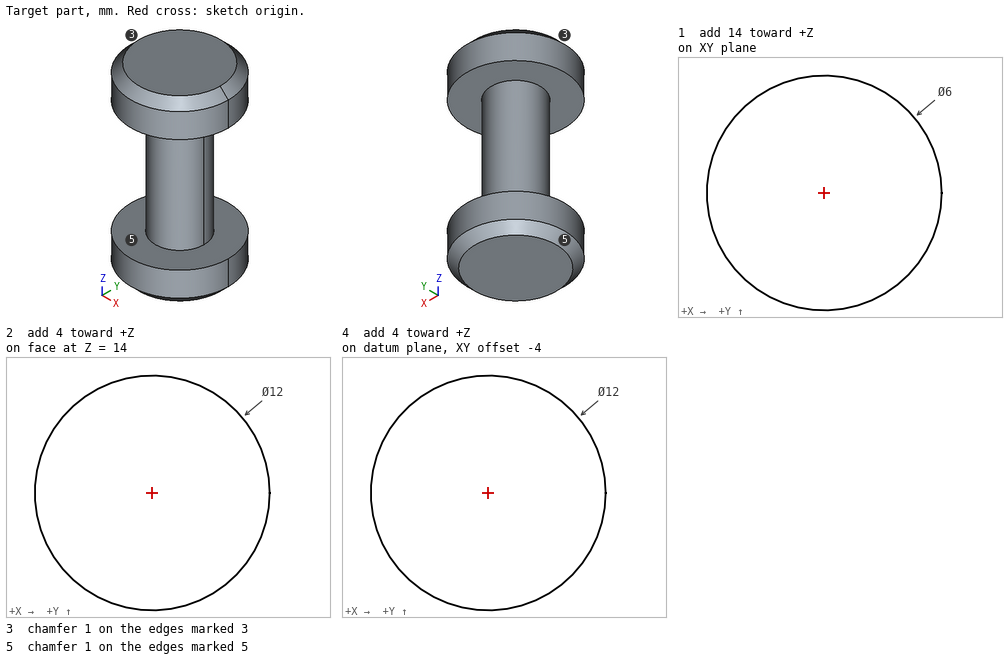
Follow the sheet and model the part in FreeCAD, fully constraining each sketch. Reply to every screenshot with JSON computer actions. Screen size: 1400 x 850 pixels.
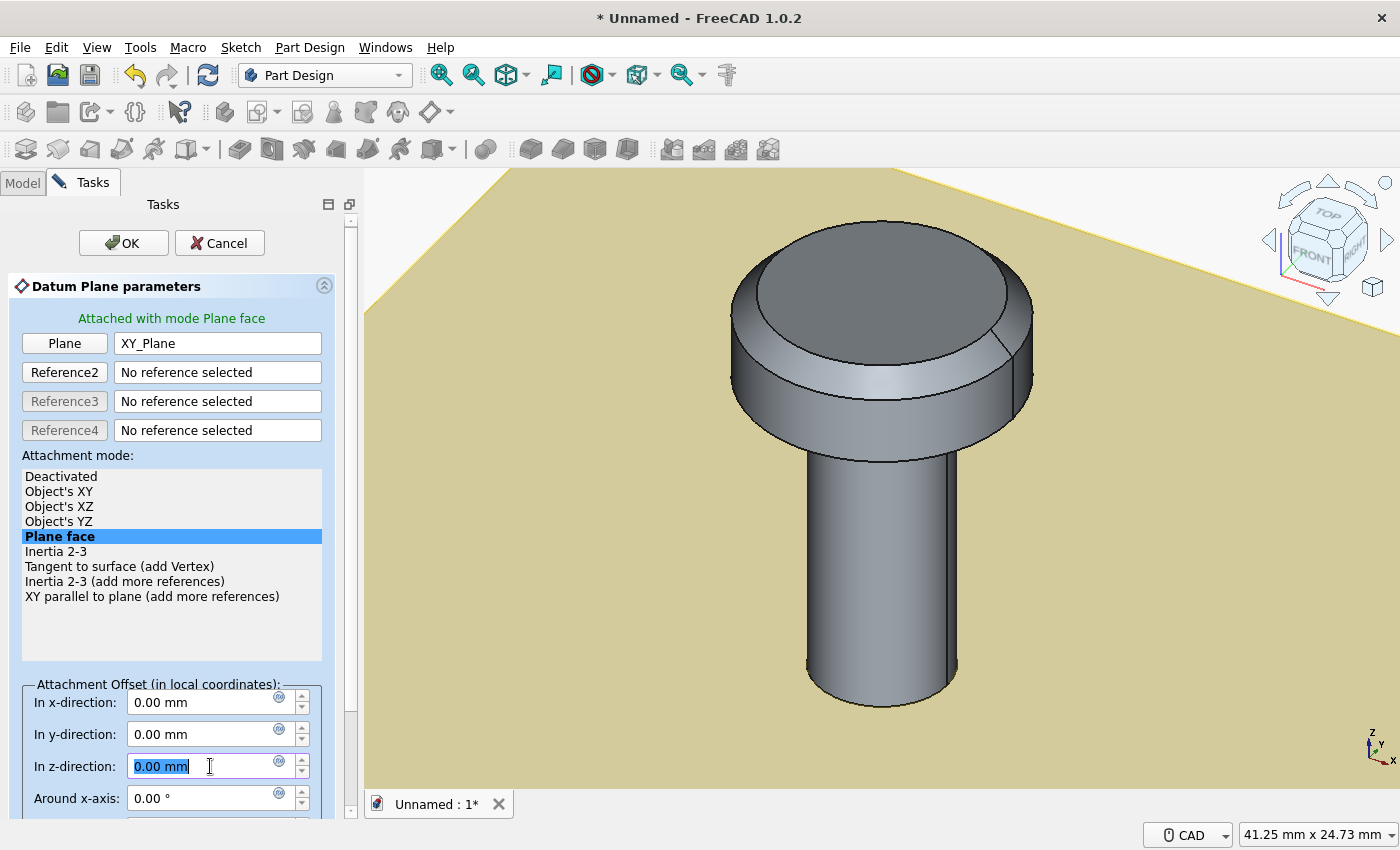
{"action": "type", "text": "-4"}
{"action": "key", "text": "Tab"}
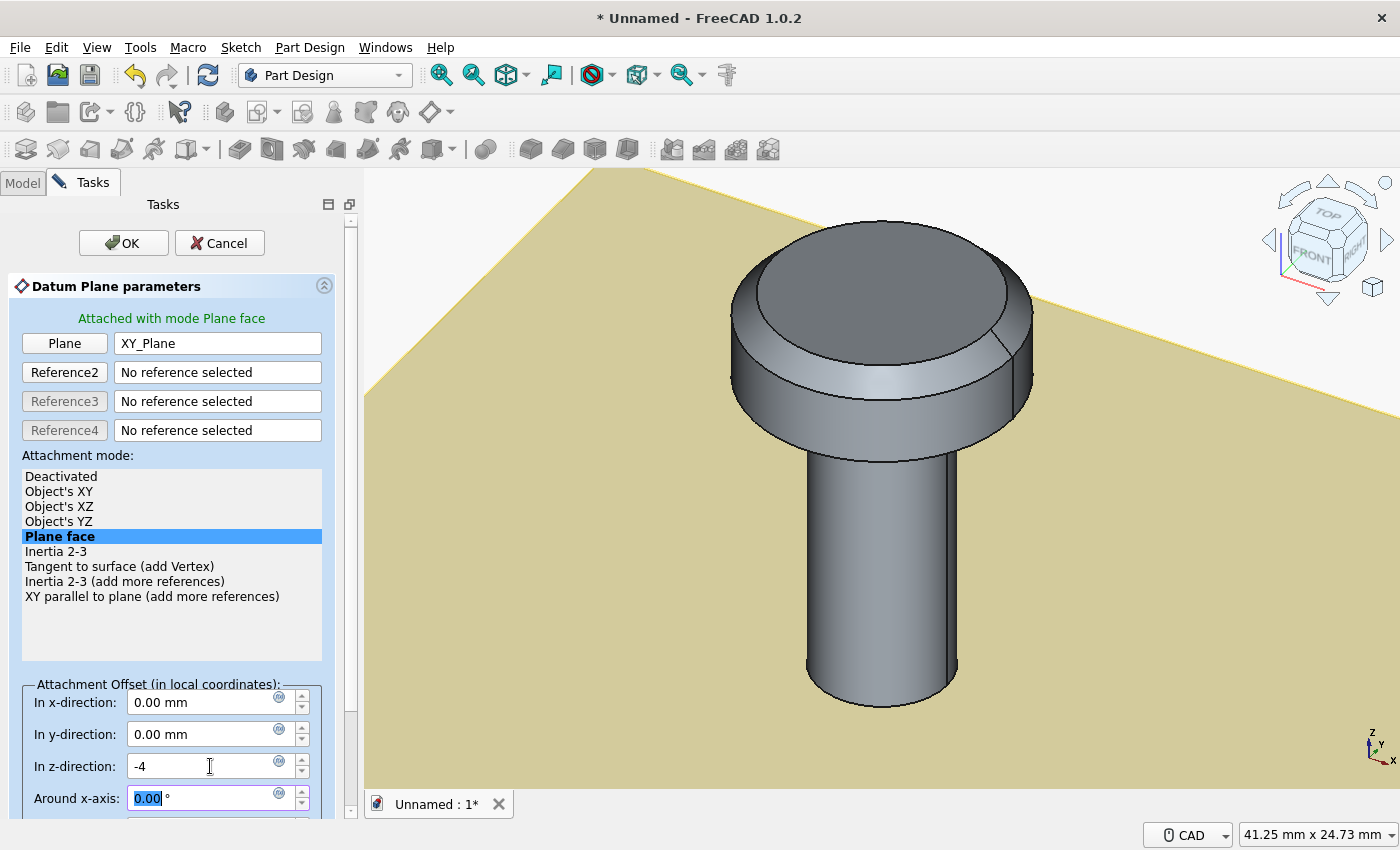
{"action": "left_click", "coordinate": [124, 243]}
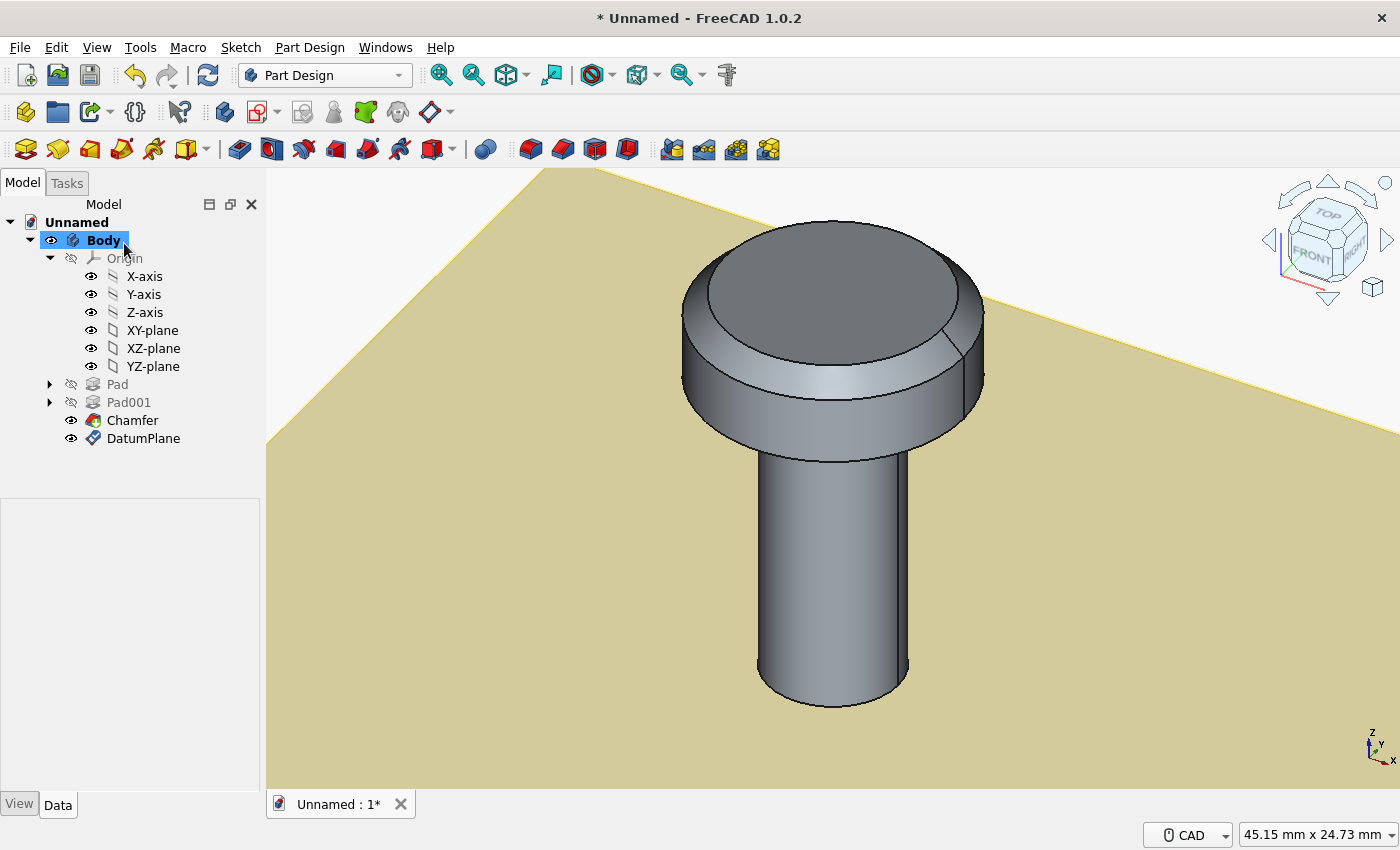
{"action": "left_click", "coordinate": [116, 438]}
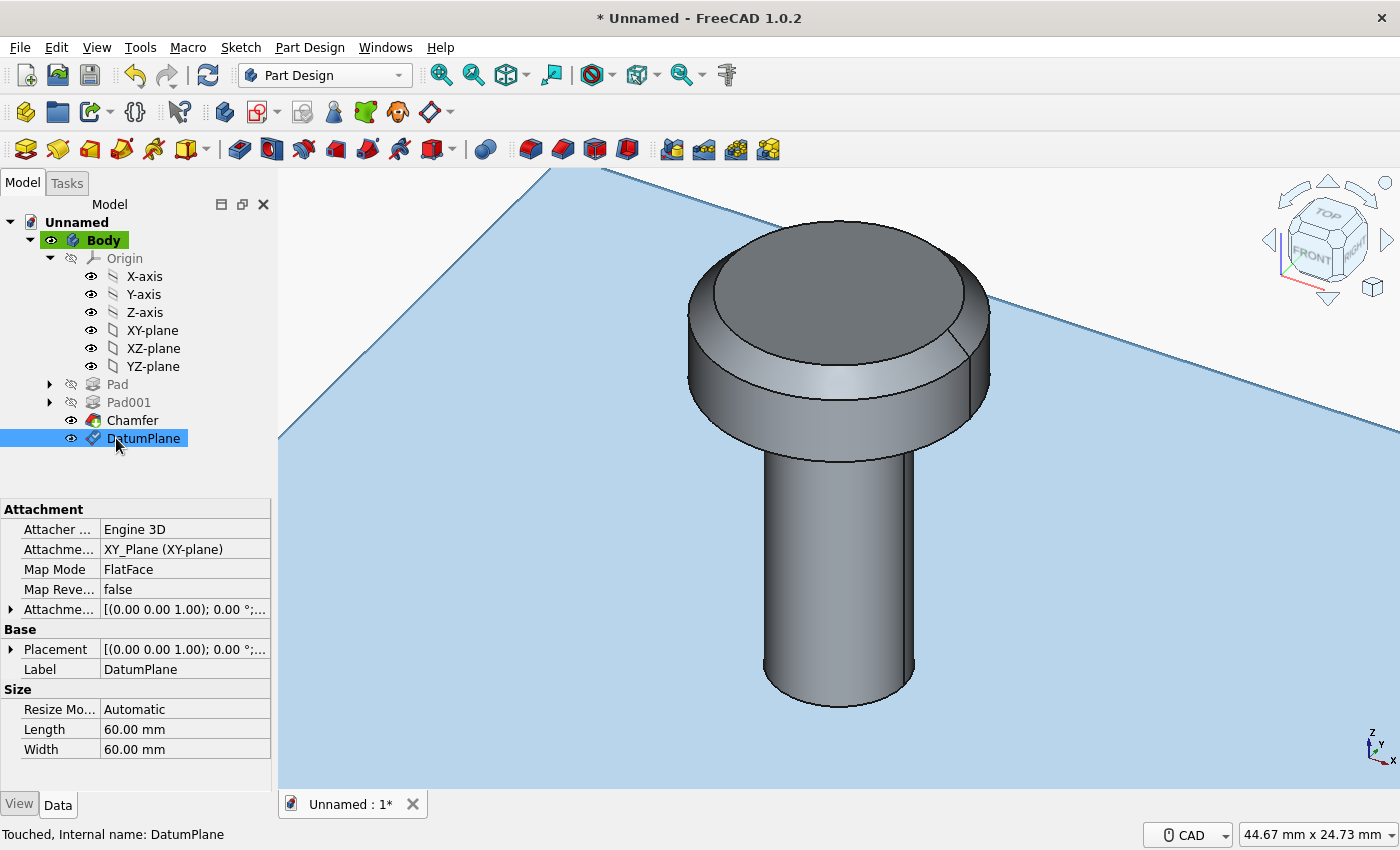
{"action": "left_click", "coordinate": [258, 112]}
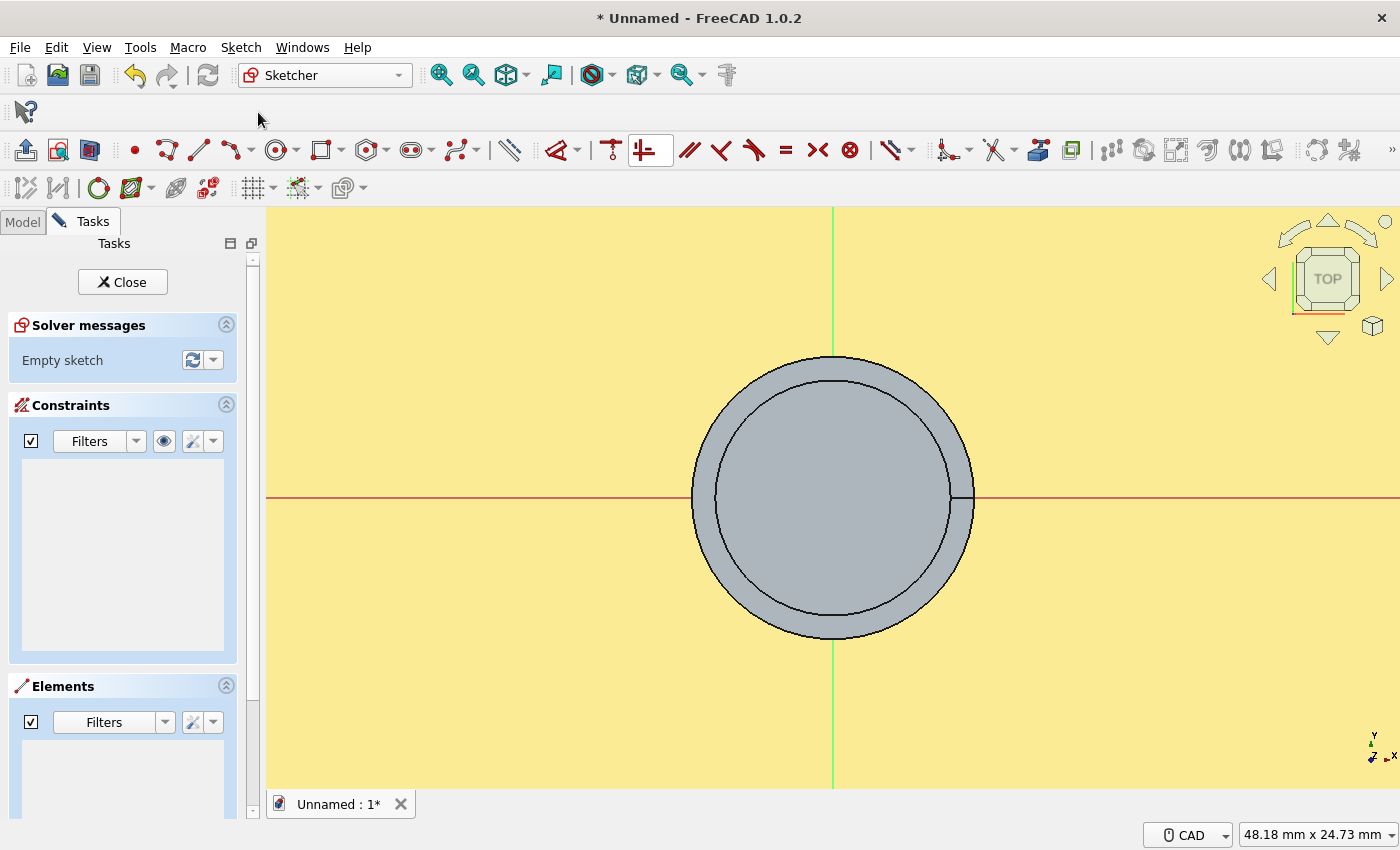
{"action": "left_click", "coordinate": [90, 150]}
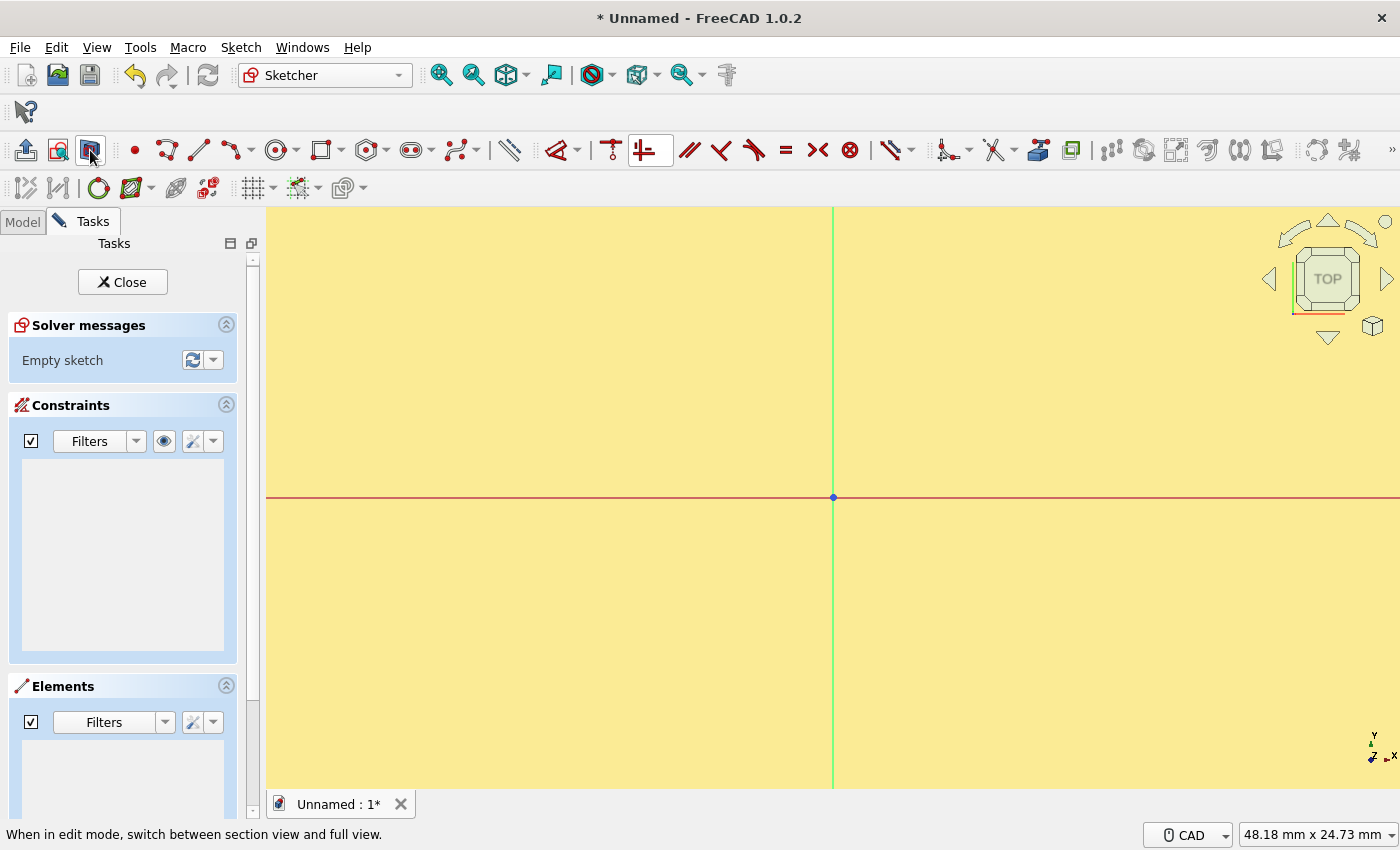
{"action": "left_click", "coordinate": [276, 150]}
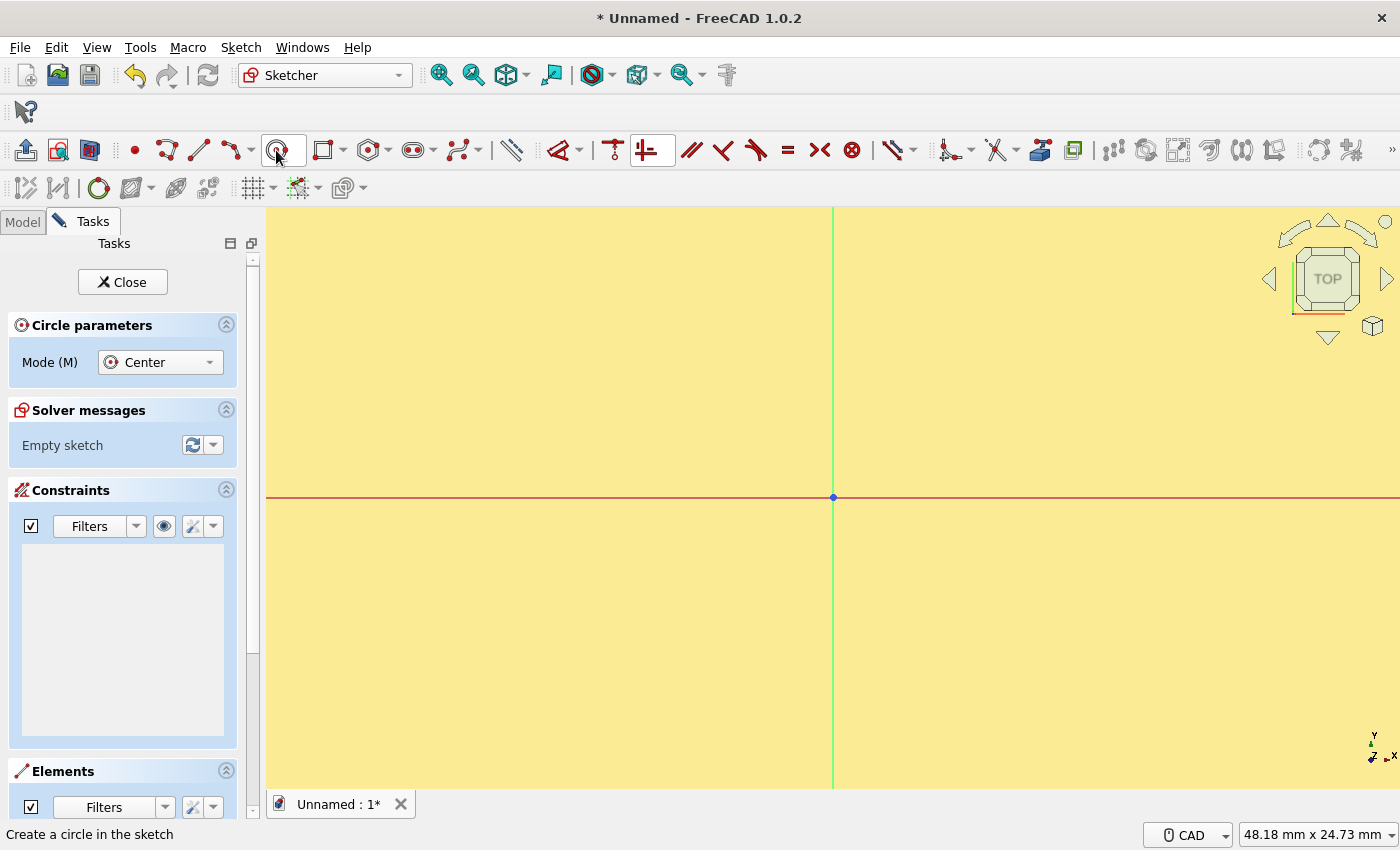
{"action": "left_click", "coordinate": [833, 498]}
{"action": "left_click", "coordinate": [933, 398]}
{"action": "key", "text": "Escape"}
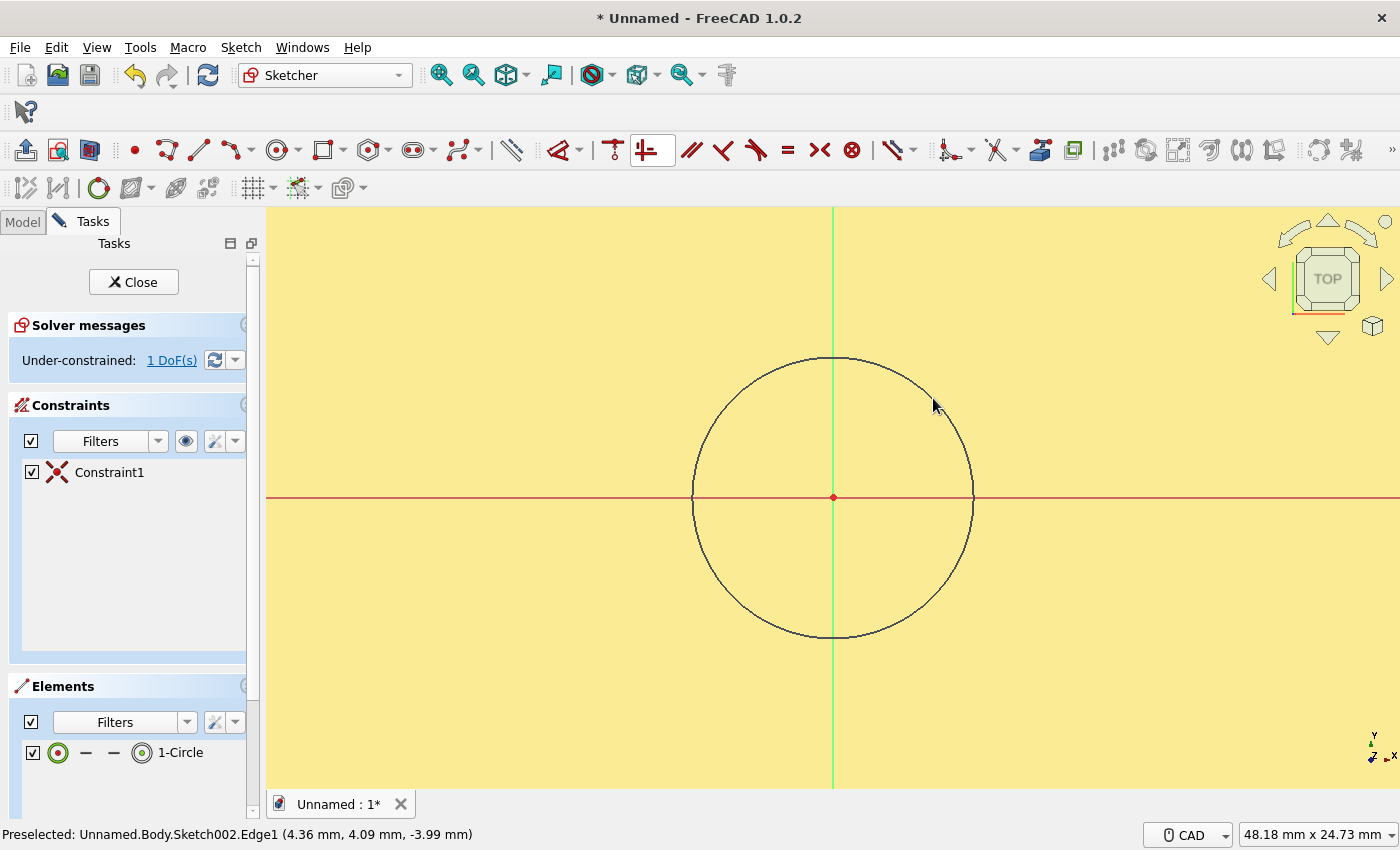
{"action": "left_click", "coordinate": [932, 398]}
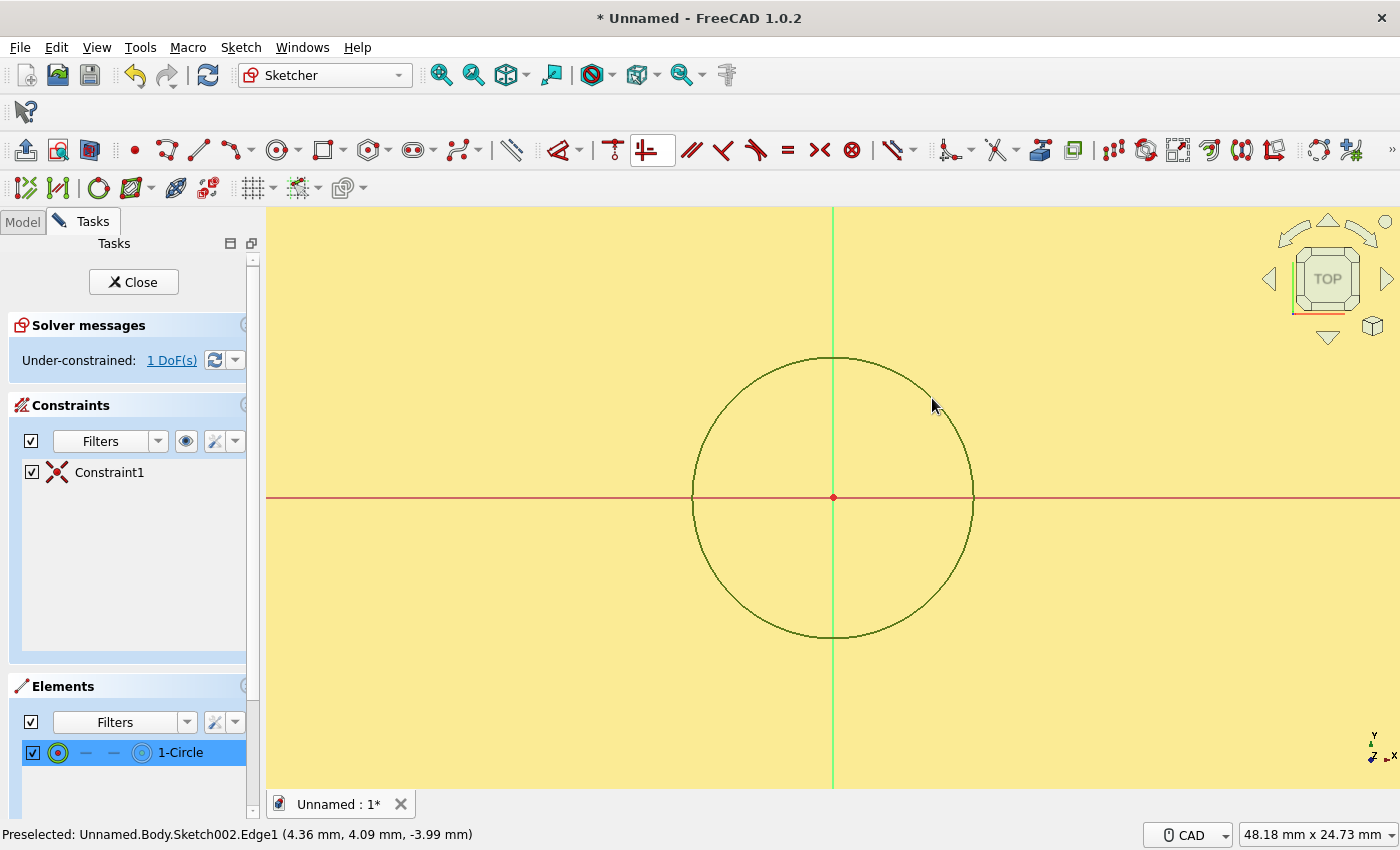
{"action": "key", "text": "k o"}